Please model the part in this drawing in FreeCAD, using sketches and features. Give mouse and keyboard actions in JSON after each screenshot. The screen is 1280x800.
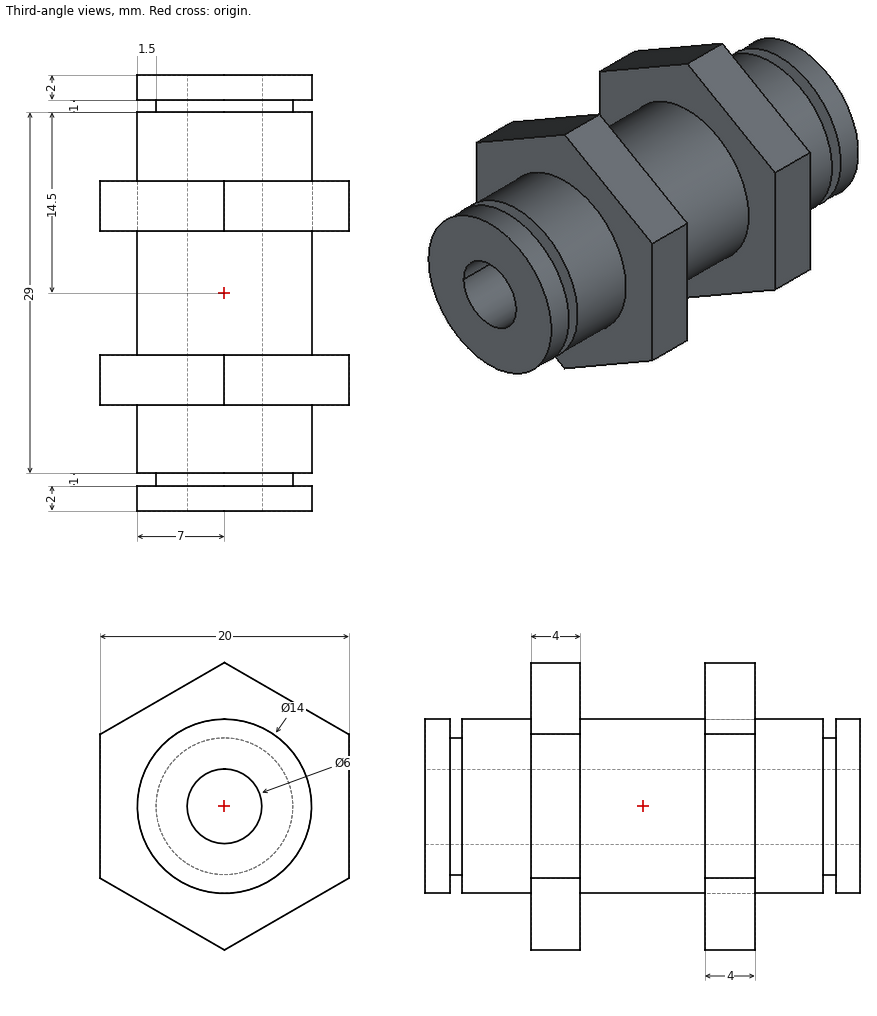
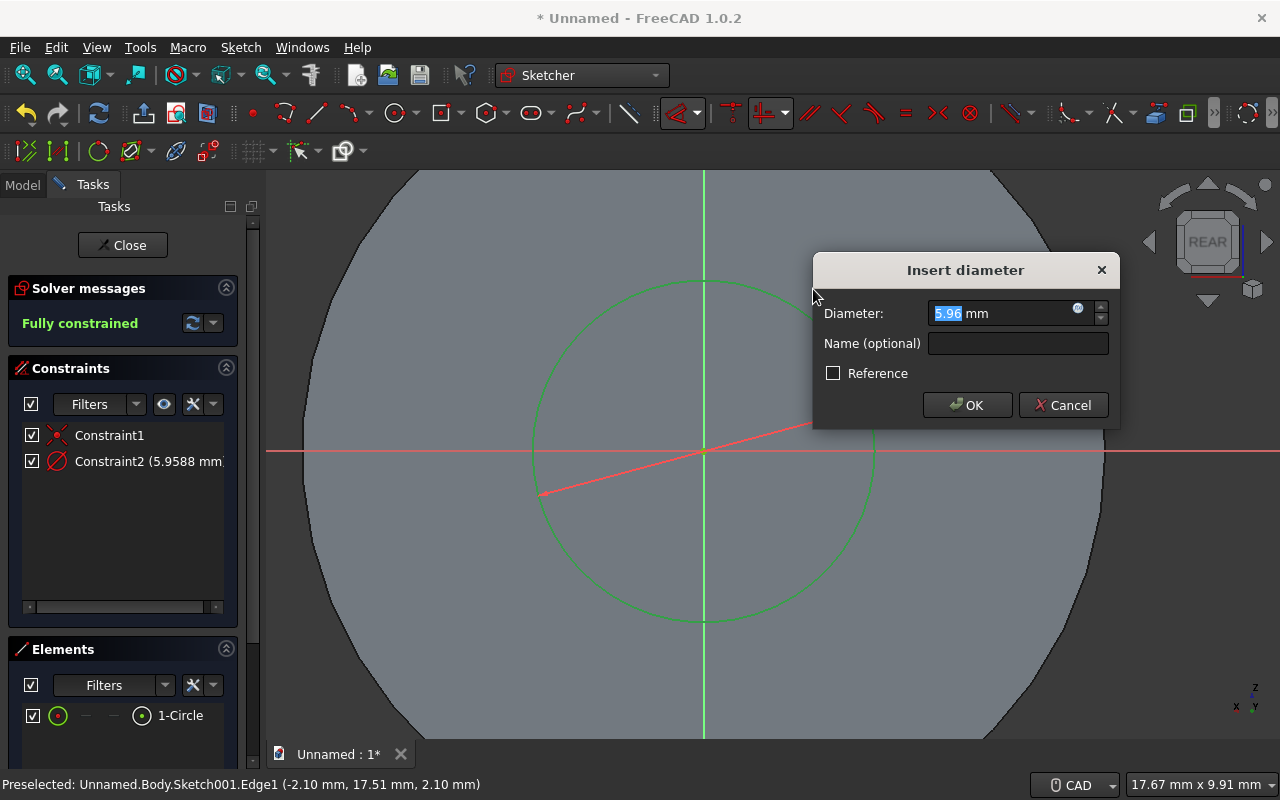
{"action": "type", "text": "6"}
{"action": "key", "text": "Return"}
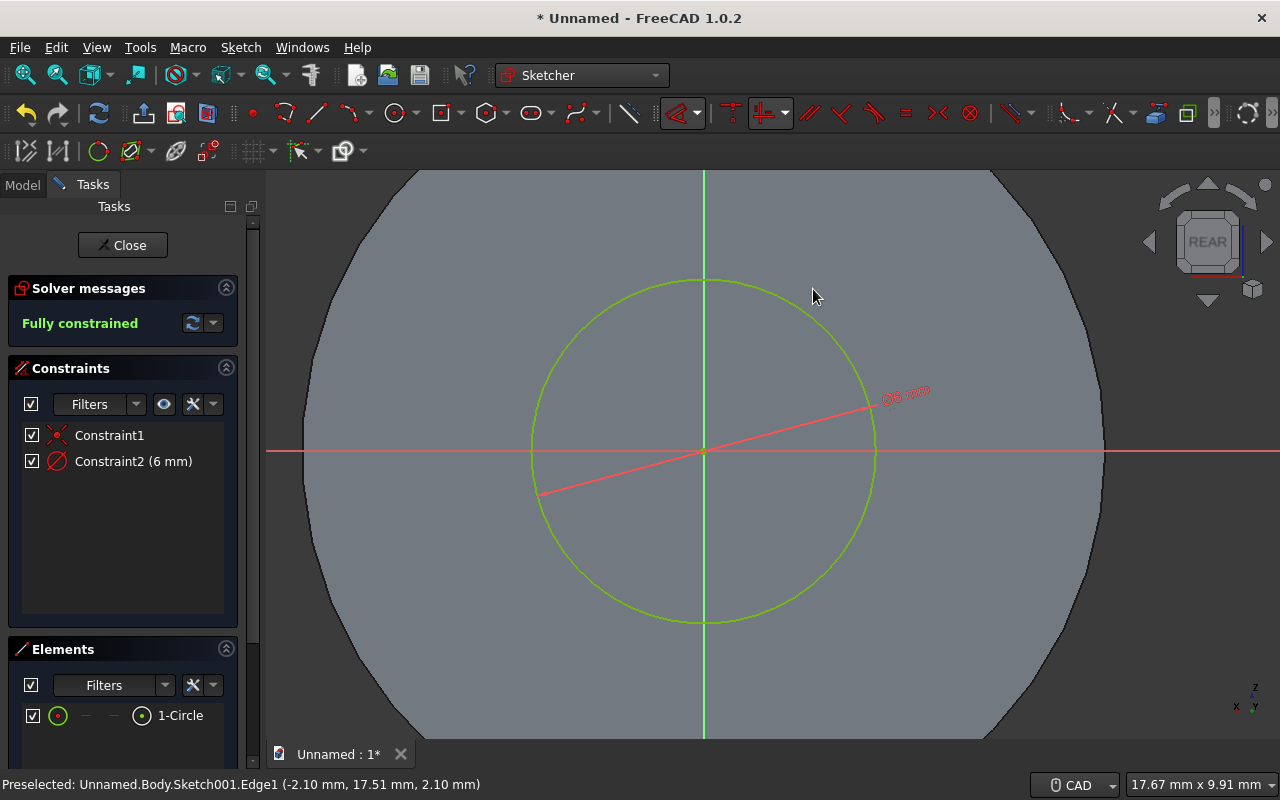
{"action": "left_click", "coordinate": [123, 245]}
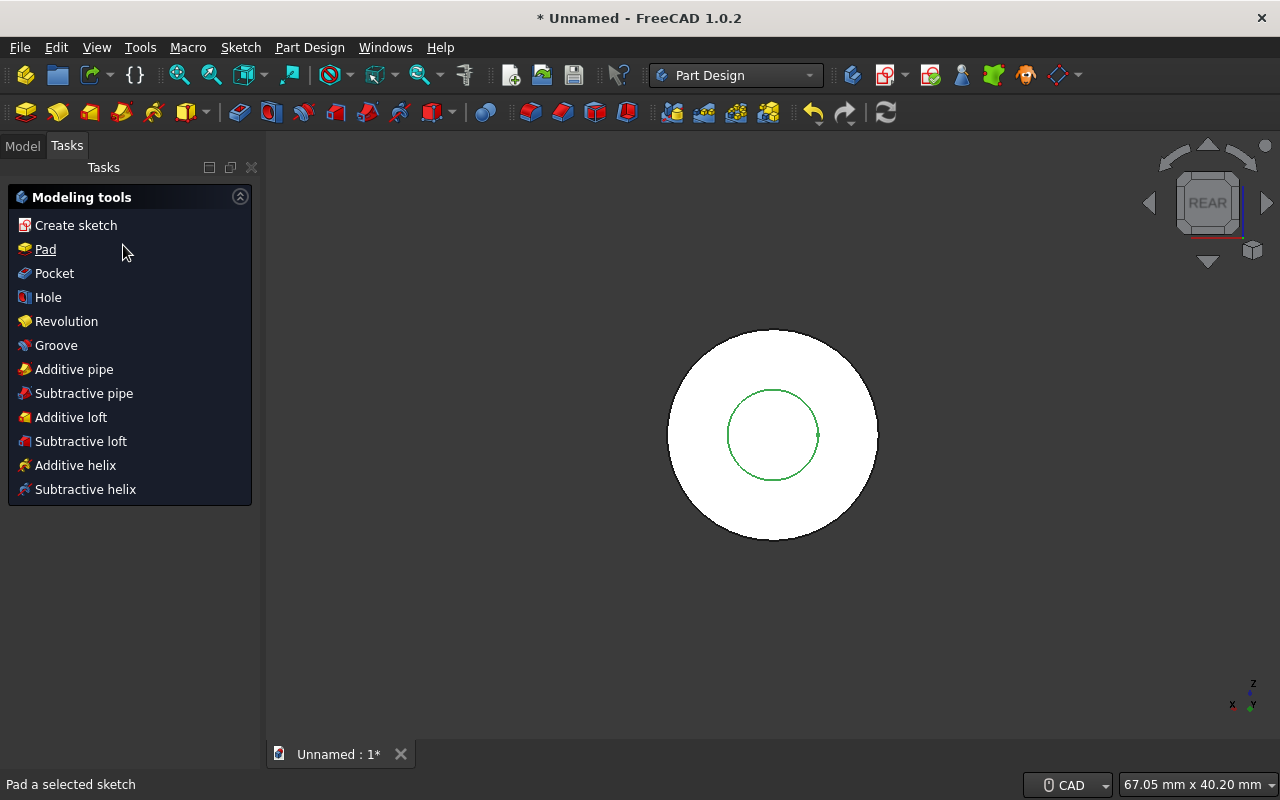
{"action": "left_click", "coordinate": [240, 112]}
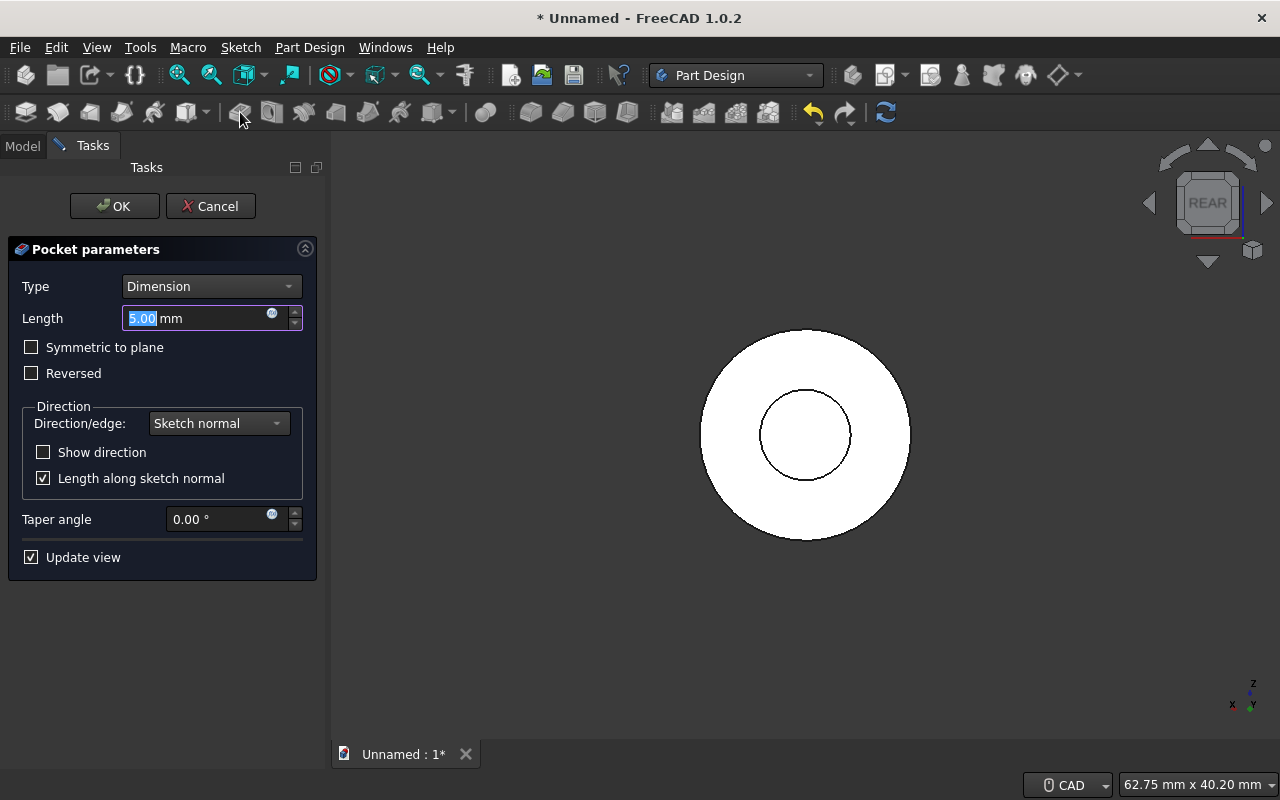
{"action": "left_click", "coordinate": [212, 286]}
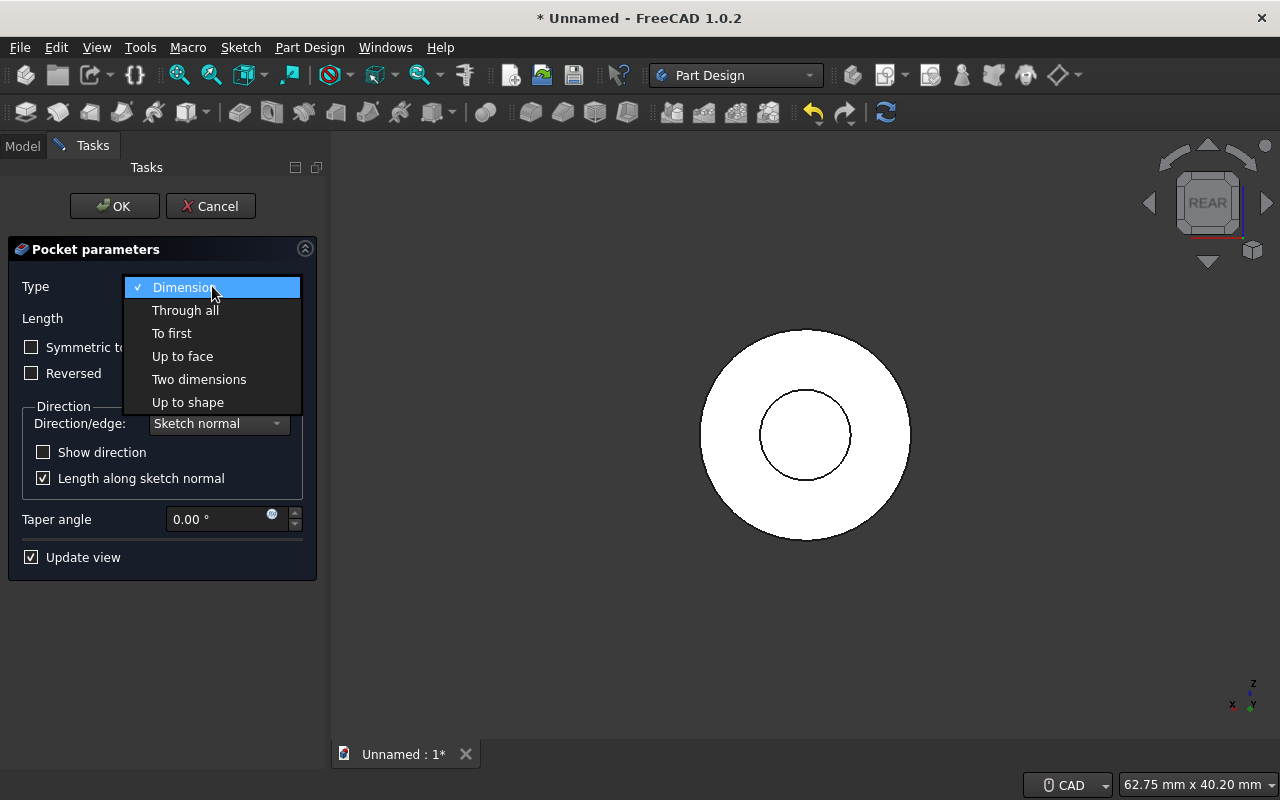
{"action": "left_click", "coordinate": [212, 310]}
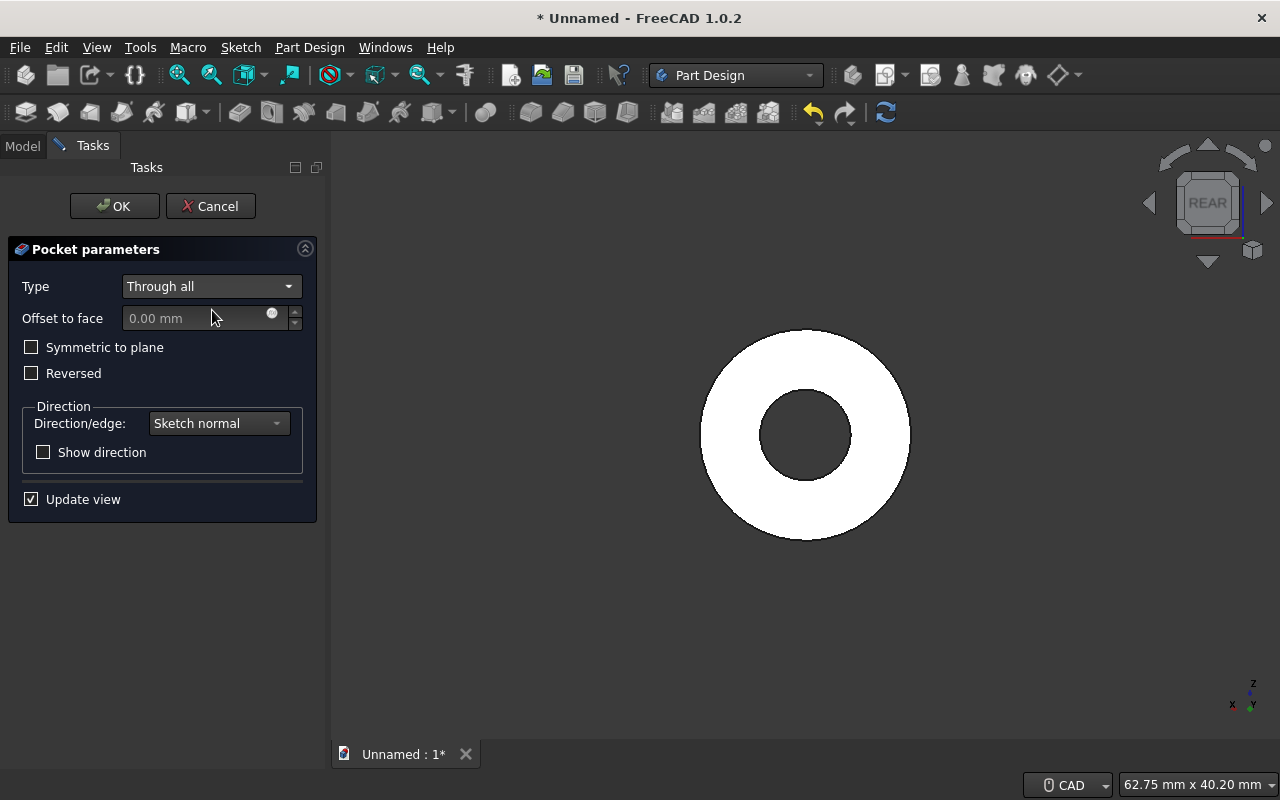
{"action": "left_click", "coordinate": [115, 206]}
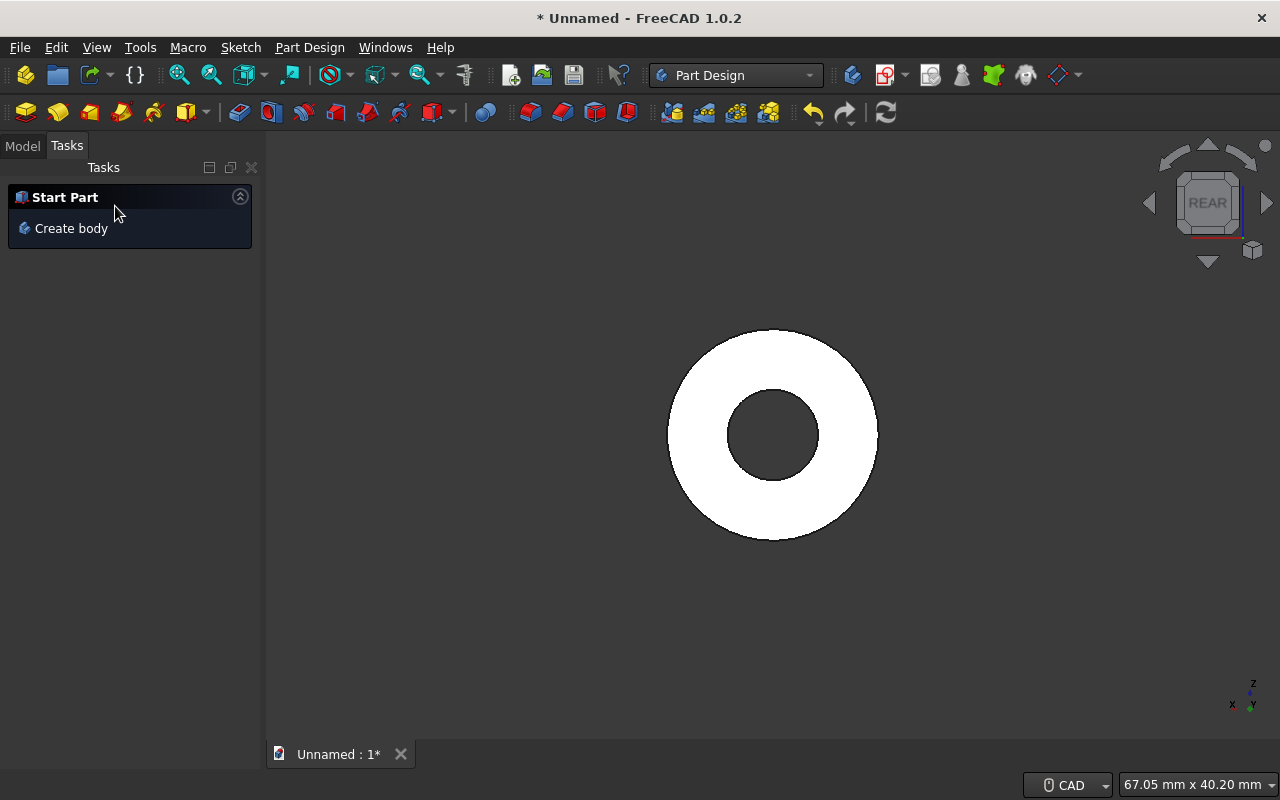
{"action": "left_click", "coordinate": [180, 76]}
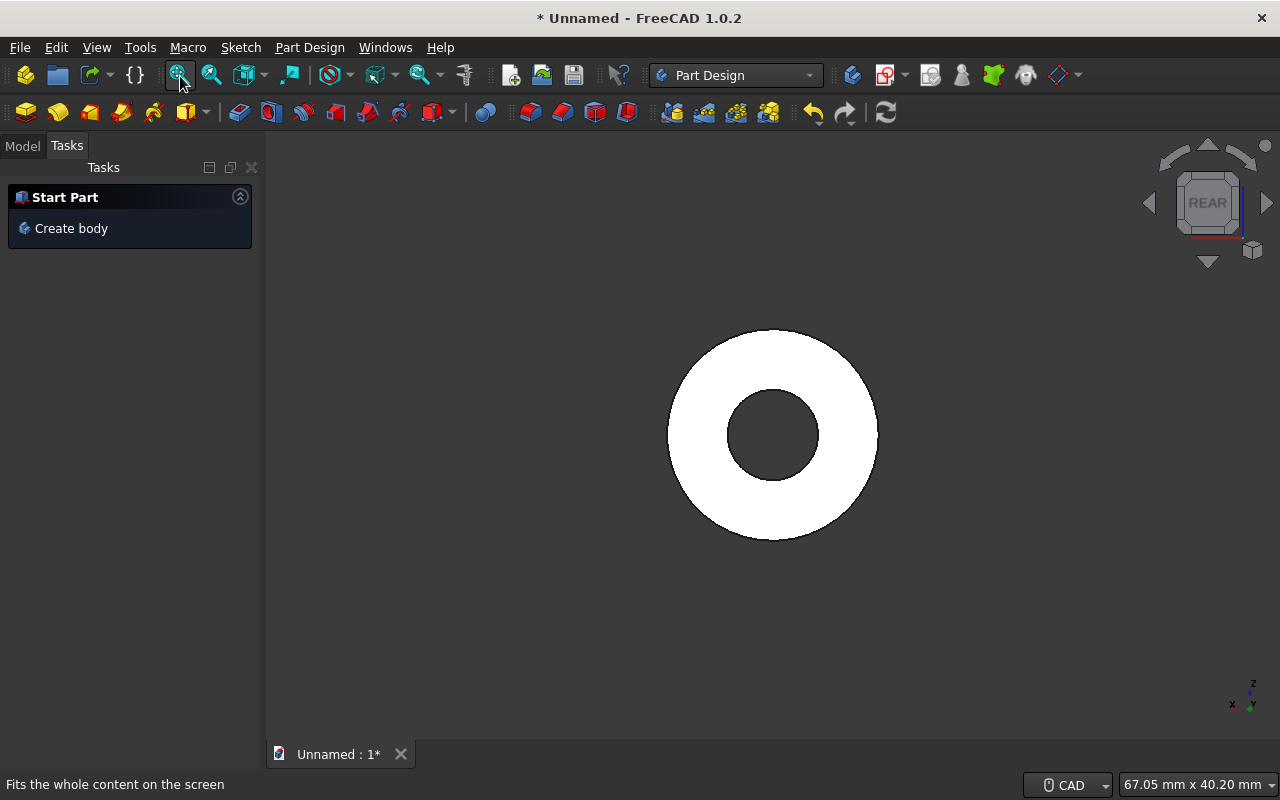
{"action": "left_click", "coordinate": [23, 145]}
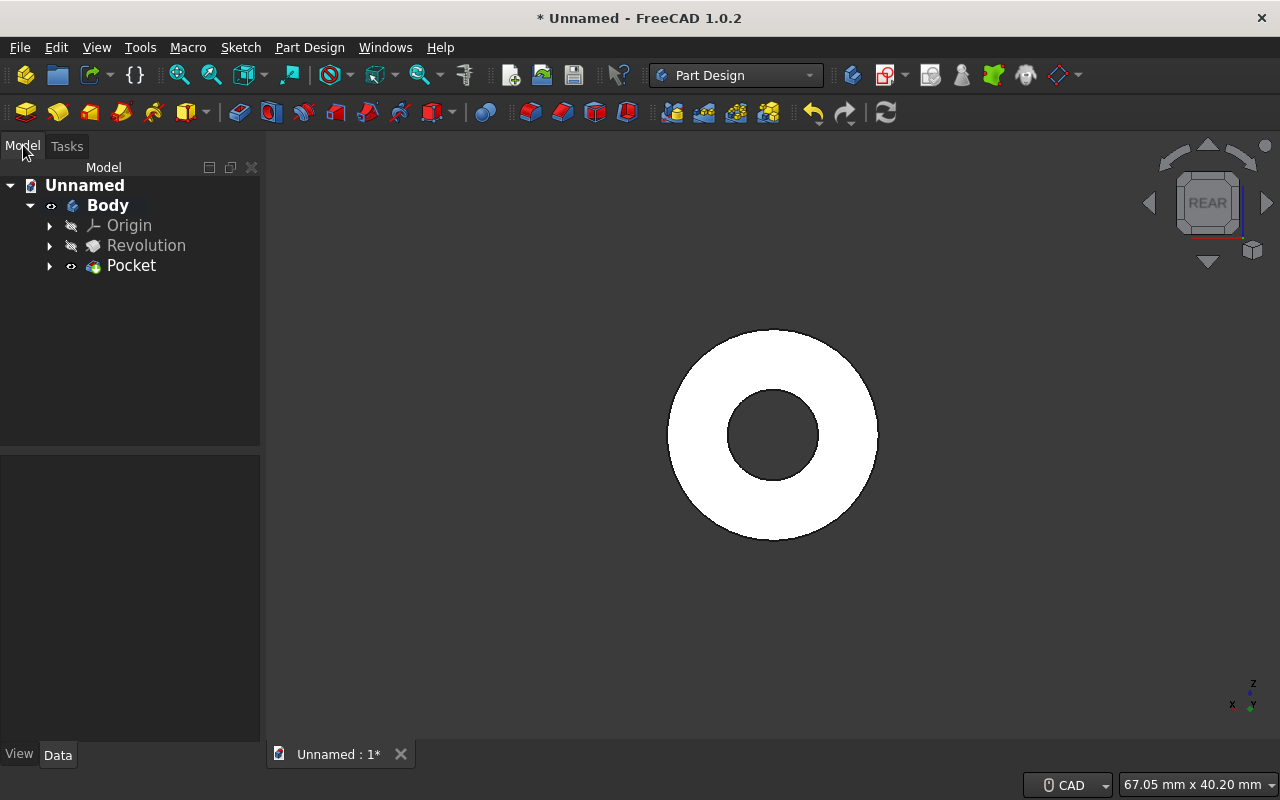
{"action": "left_click", "coordinate": [50, 226]}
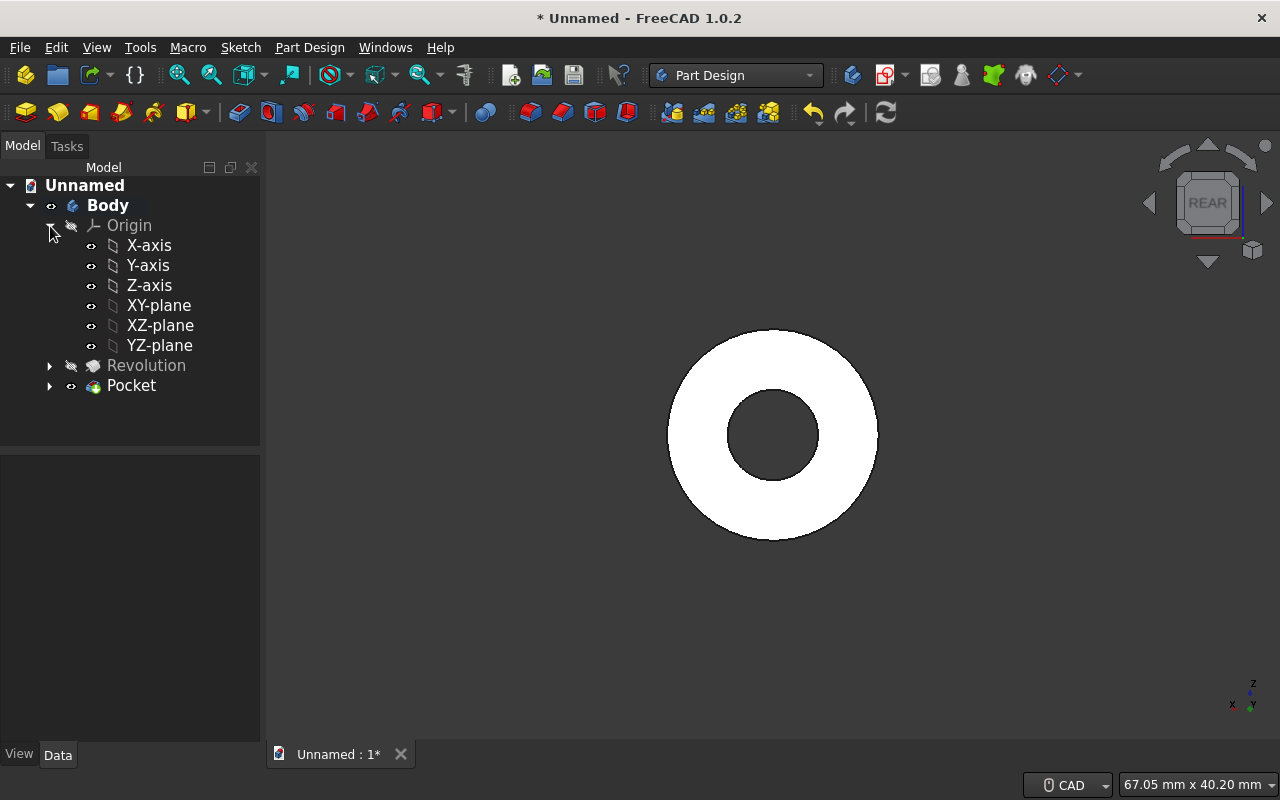
{"action": "left_click", "coordinate": [136, 326]}